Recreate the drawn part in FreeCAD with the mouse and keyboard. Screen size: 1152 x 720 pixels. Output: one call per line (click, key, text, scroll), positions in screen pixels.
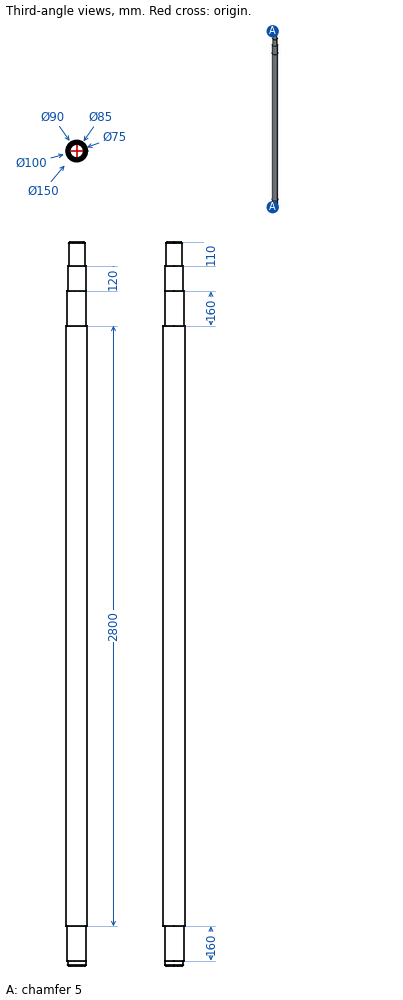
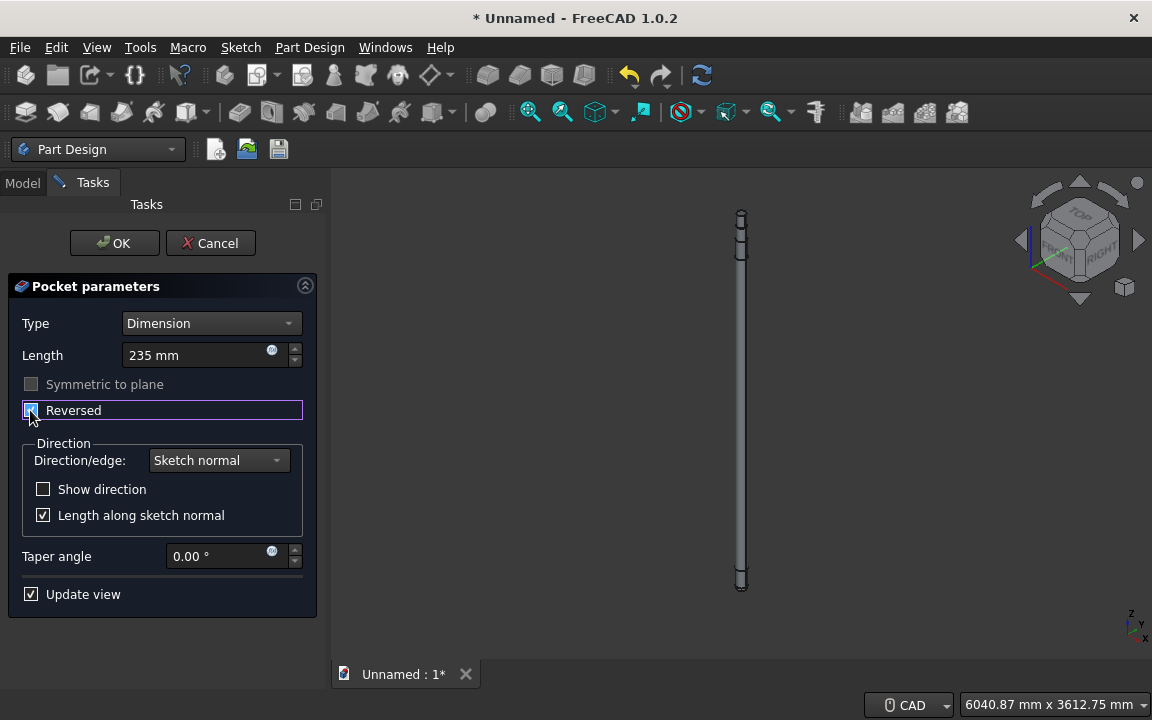
click(115, 243)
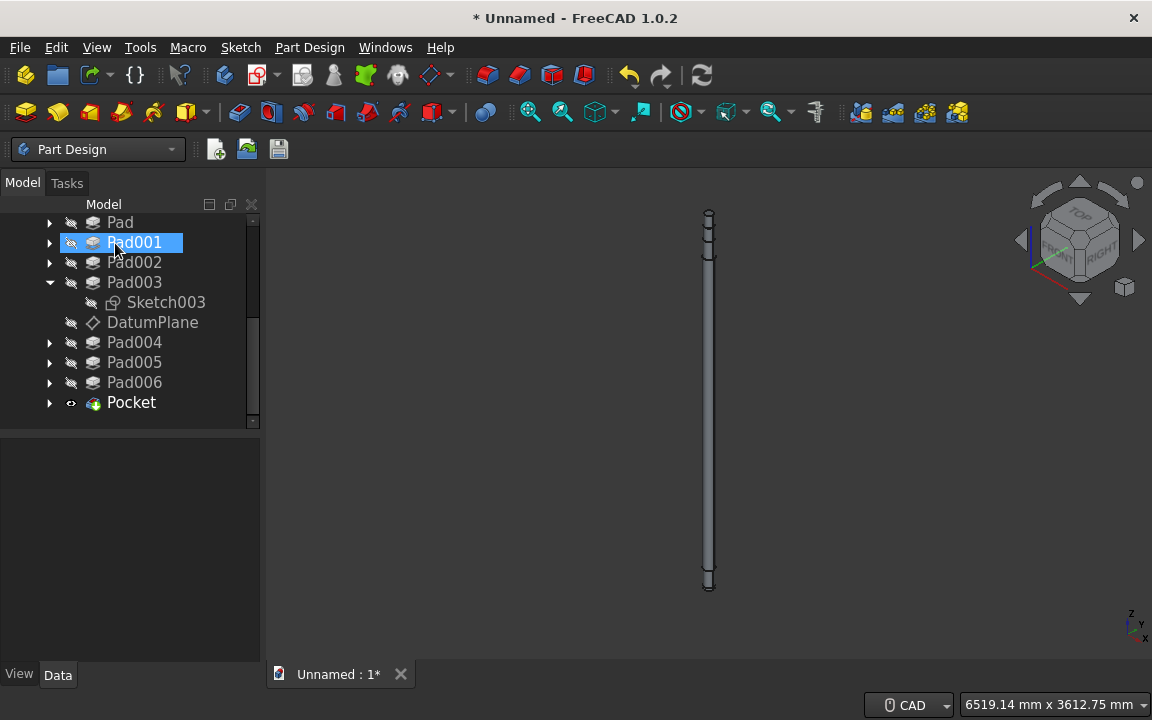
click(705, 210)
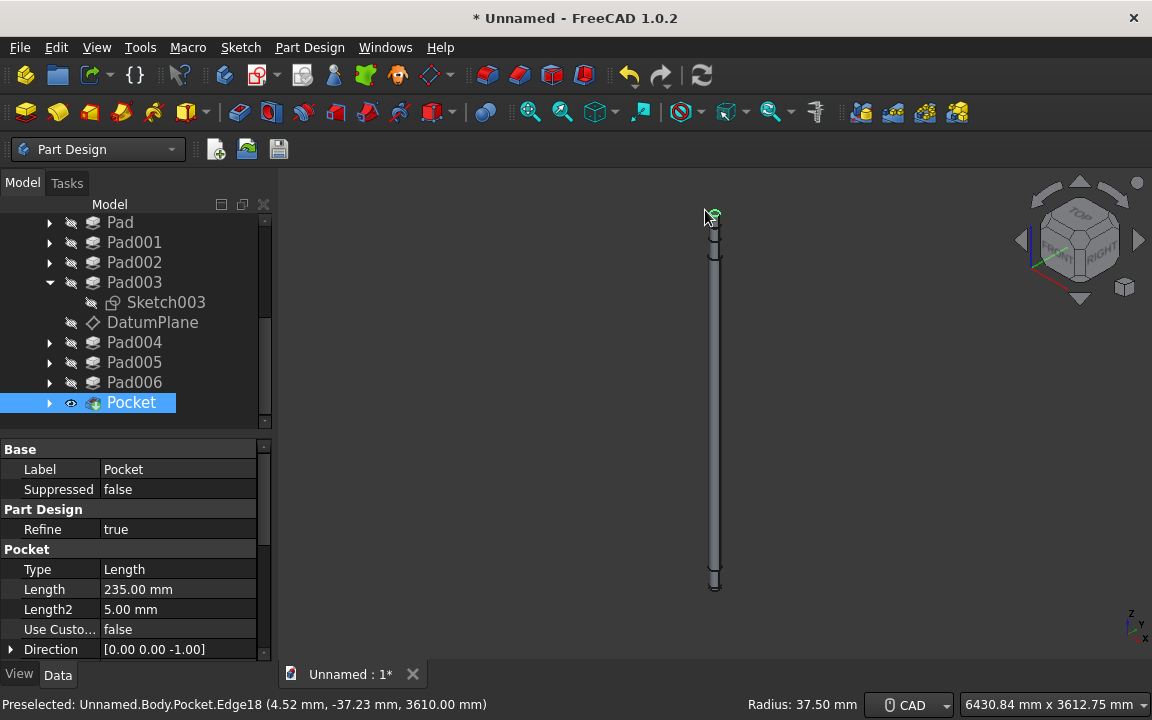
key(2)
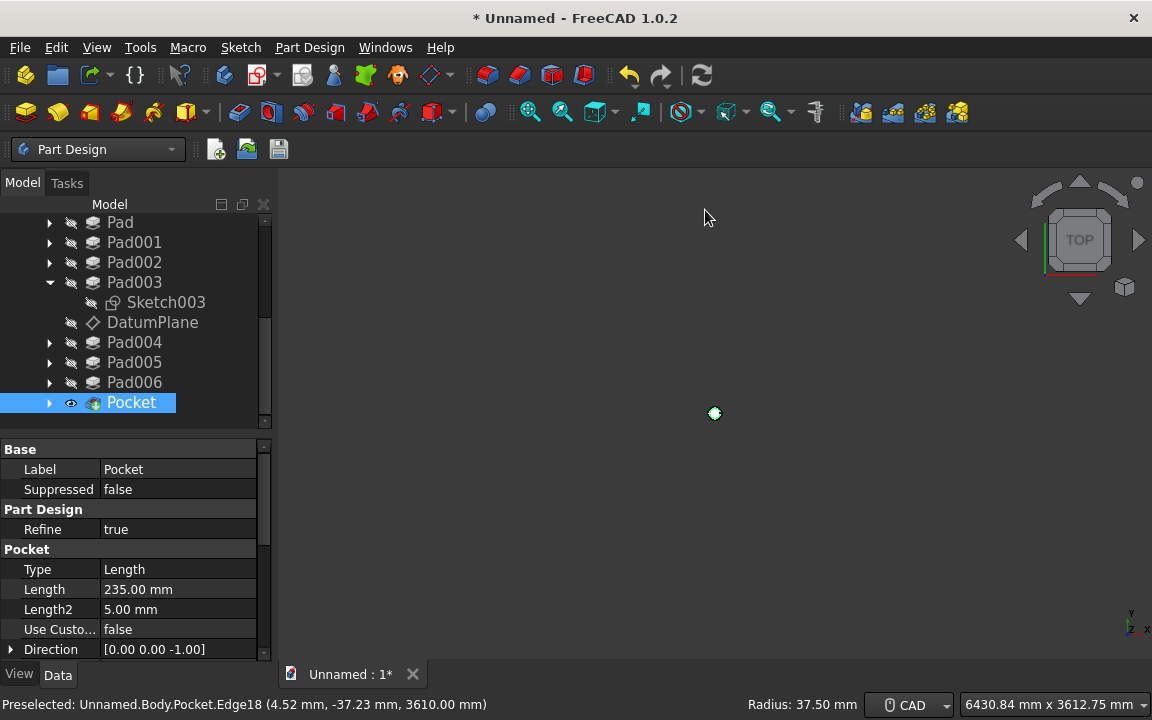
click(532, 112)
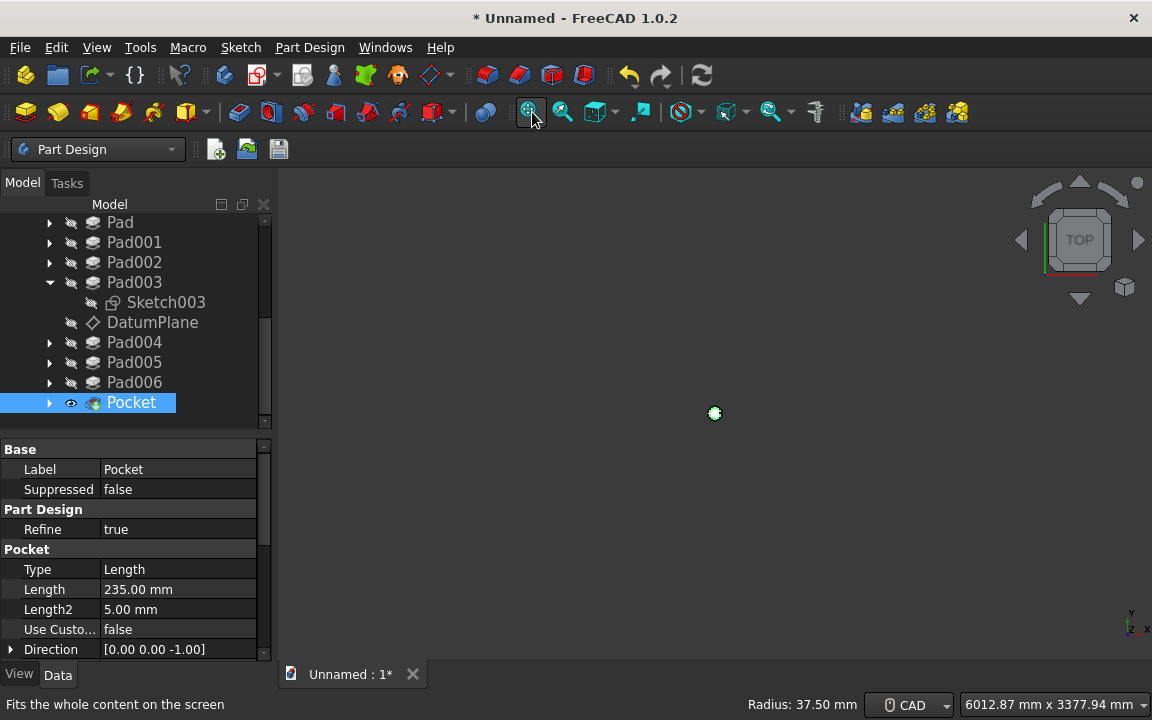
key(0)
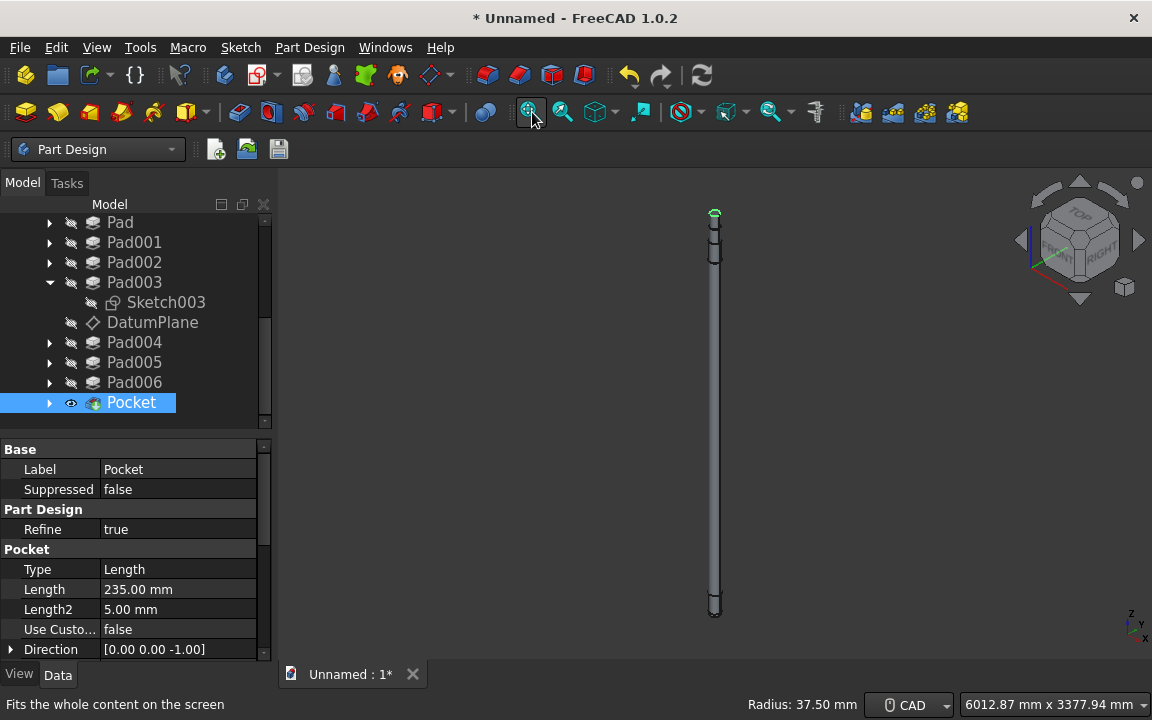
key(1)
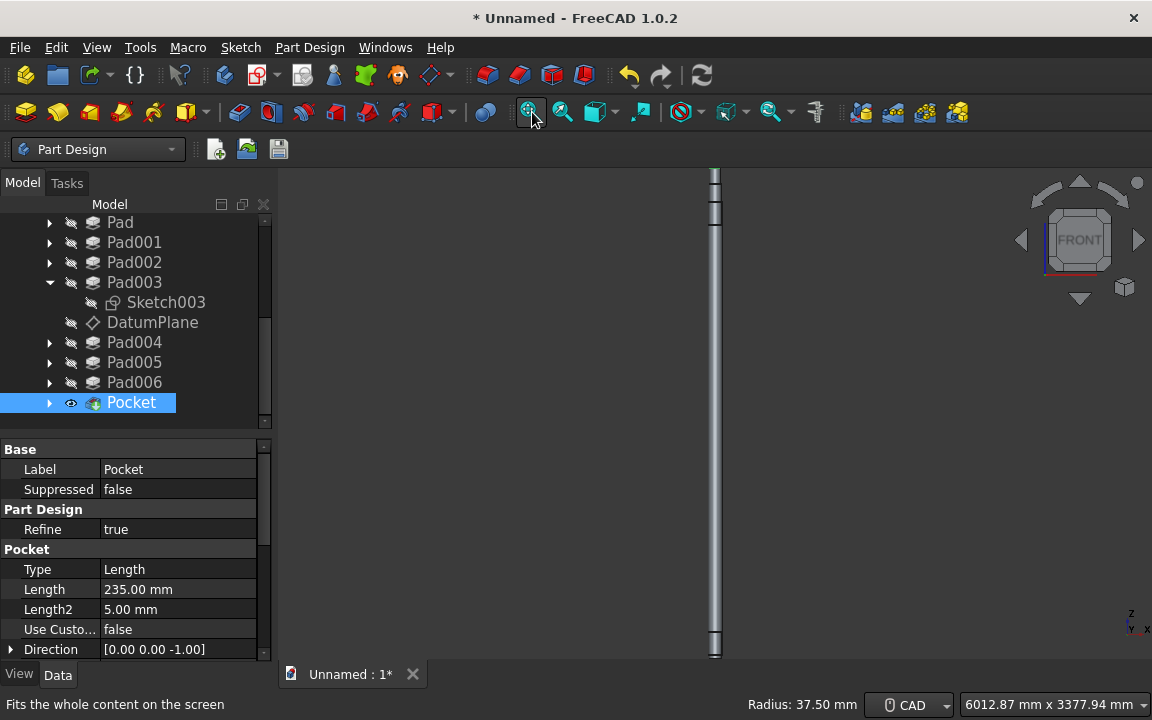
click(532, 112)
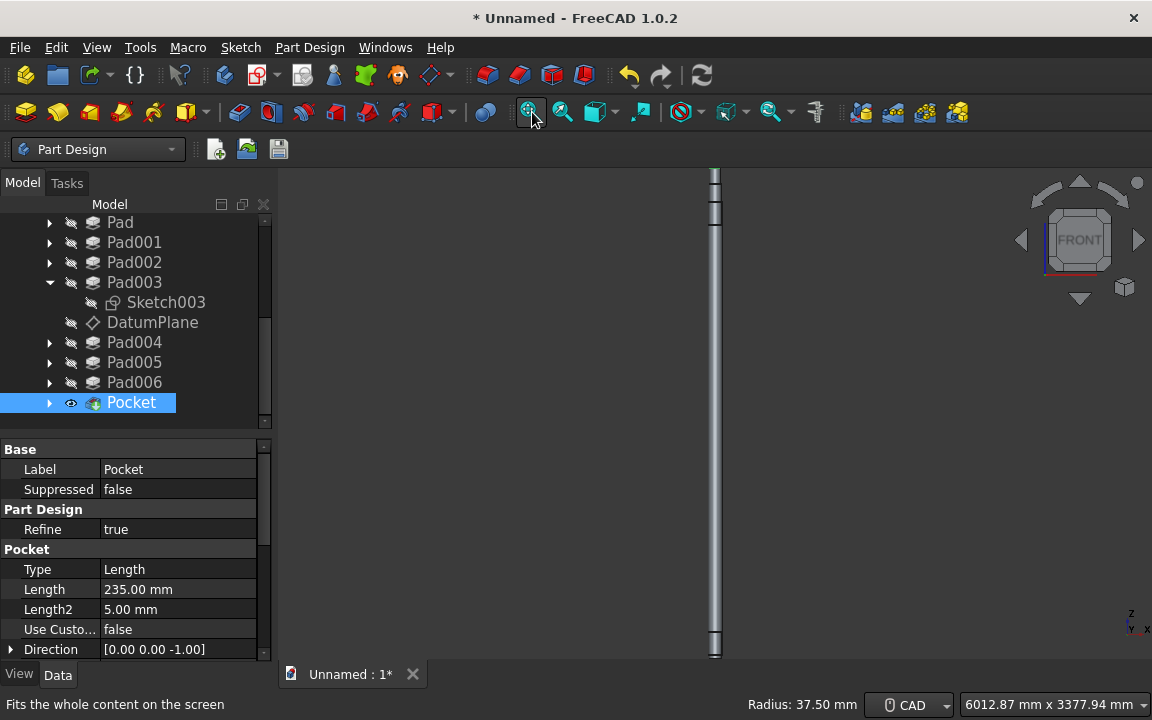
key(3)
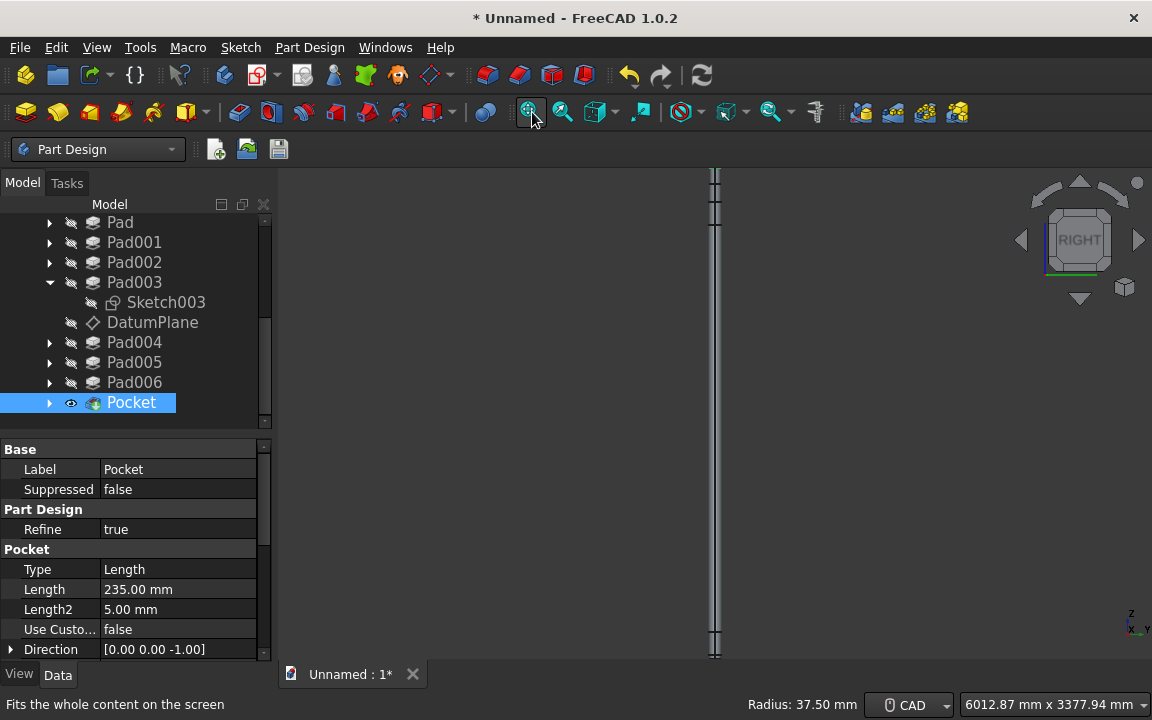
click(532, 112)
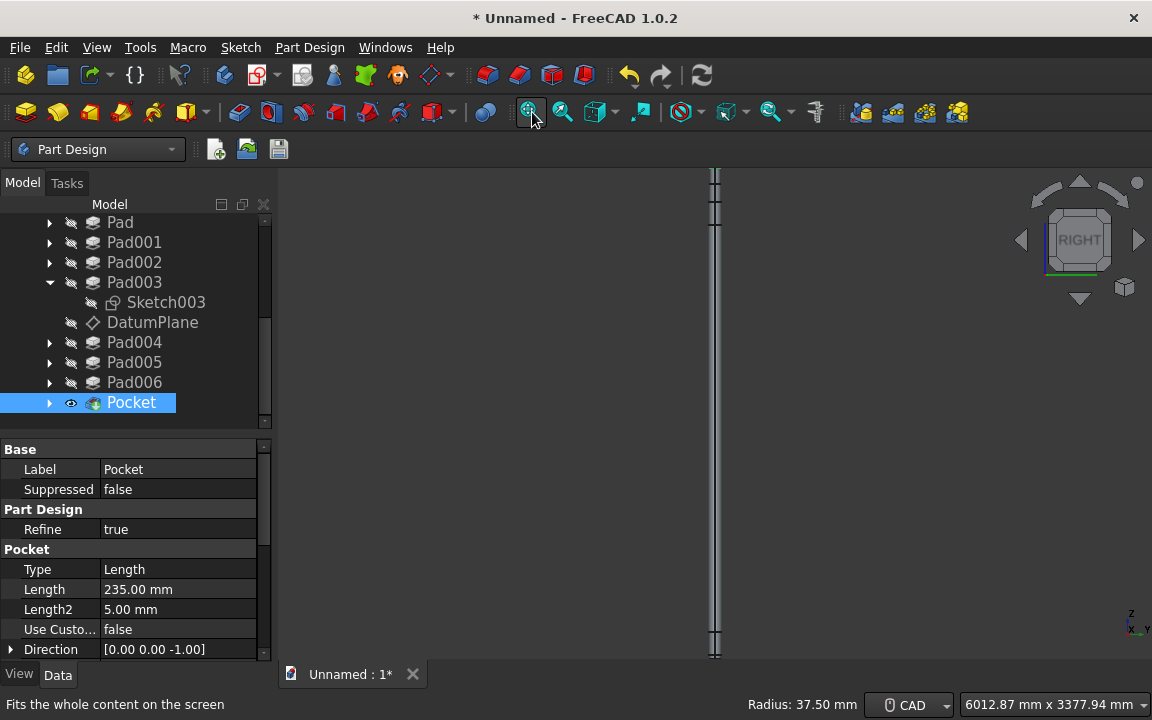
key(5)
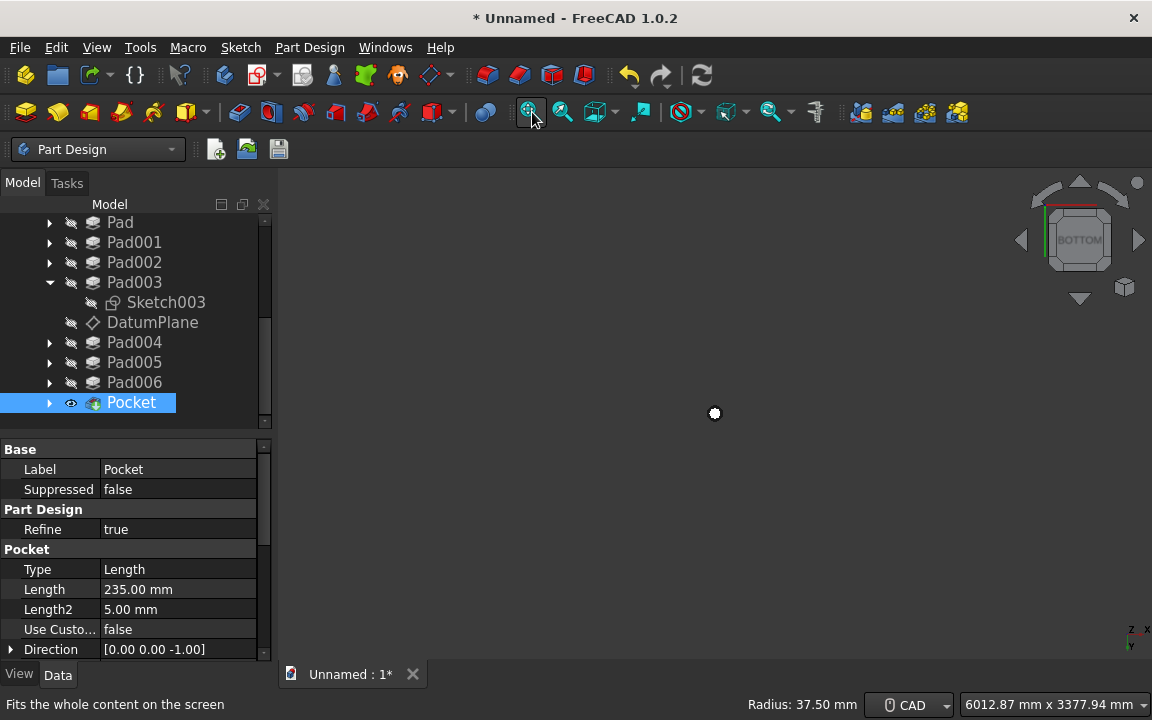
click(532, 112)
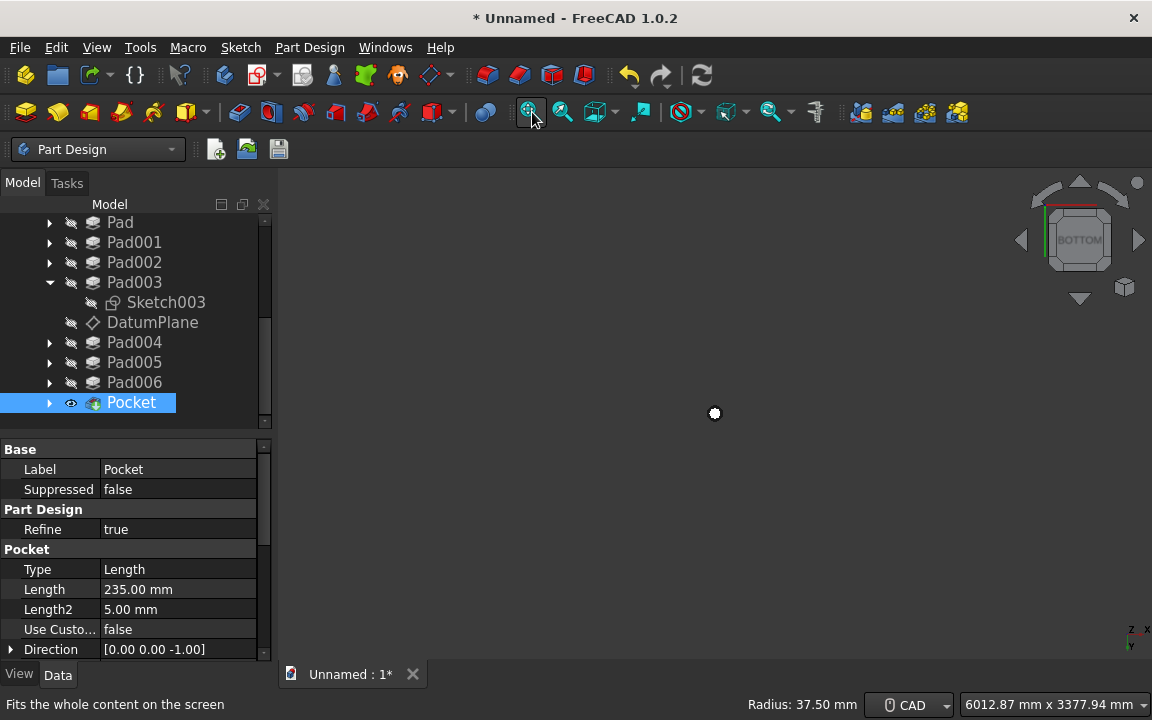
click(709, 412, ctrl)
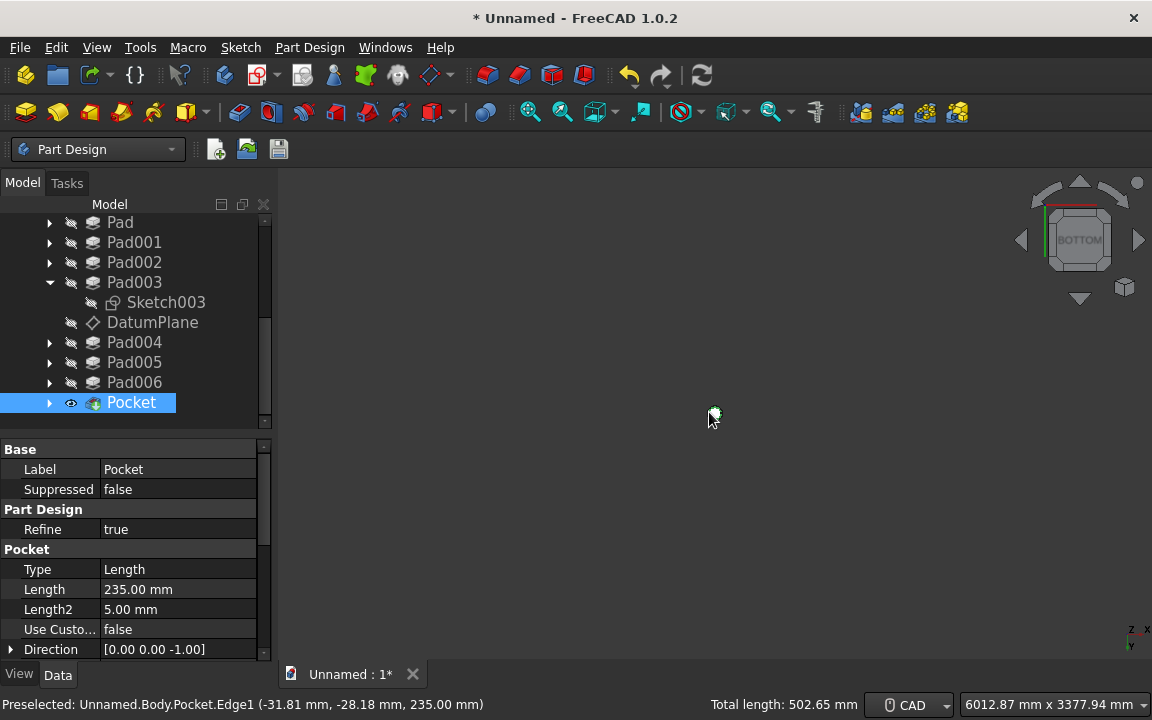
click(520, 76)